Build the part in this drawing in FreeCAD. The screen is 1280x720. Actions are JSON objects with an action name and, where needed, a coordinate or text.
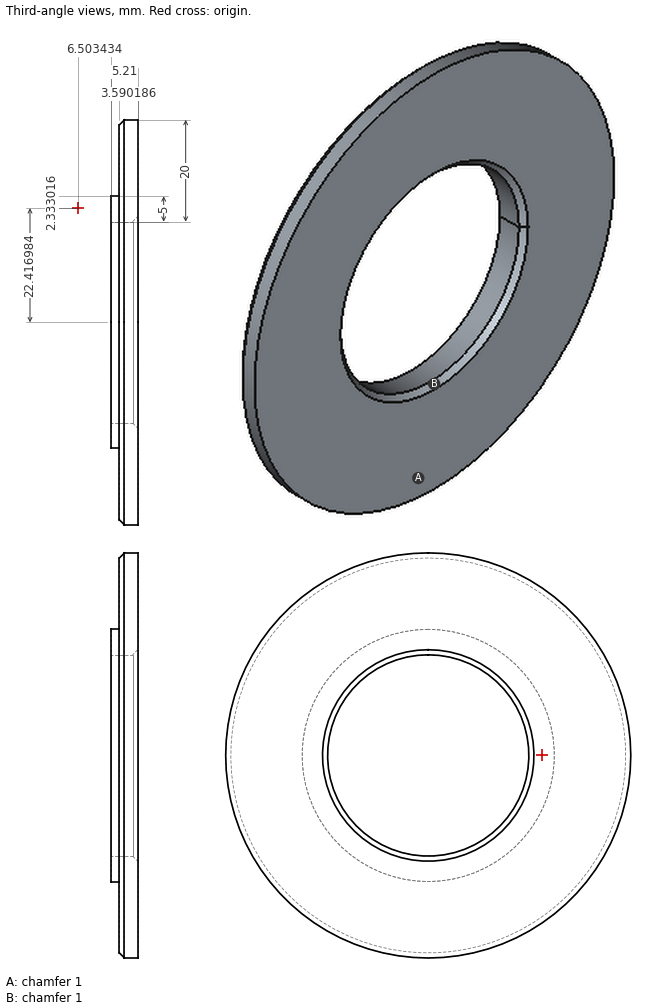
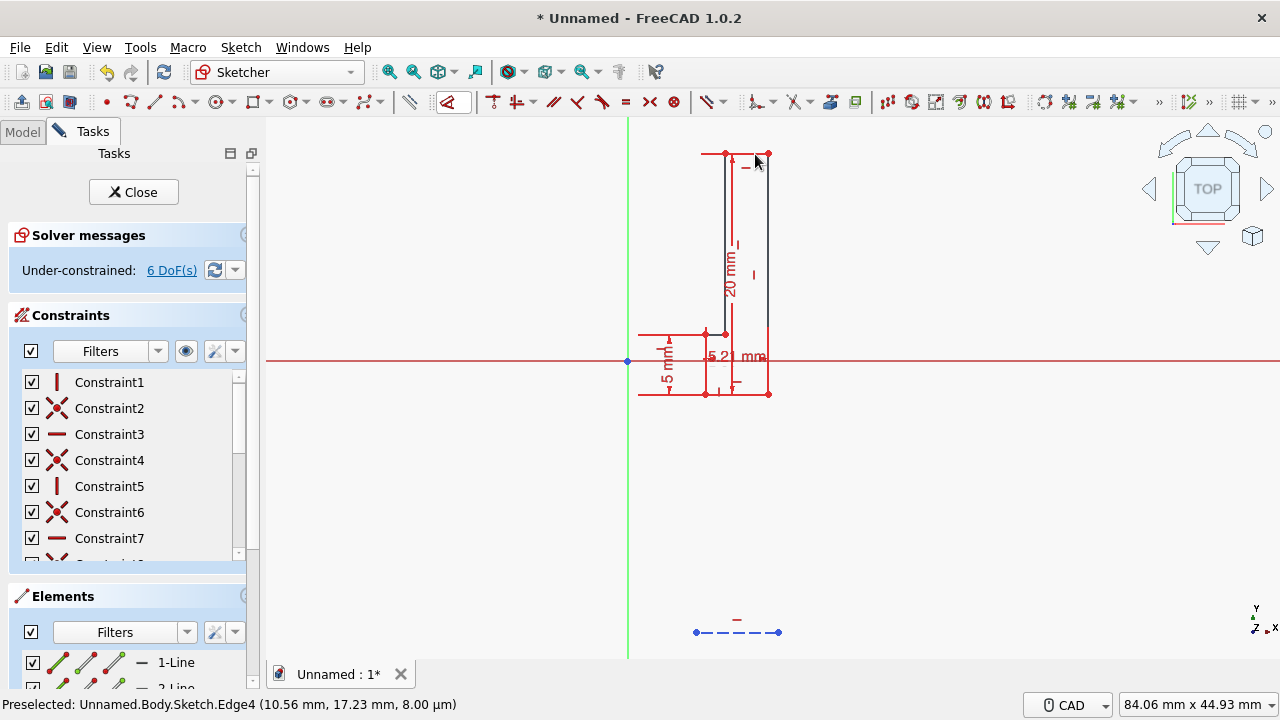
{"action": "key", "text": "l"}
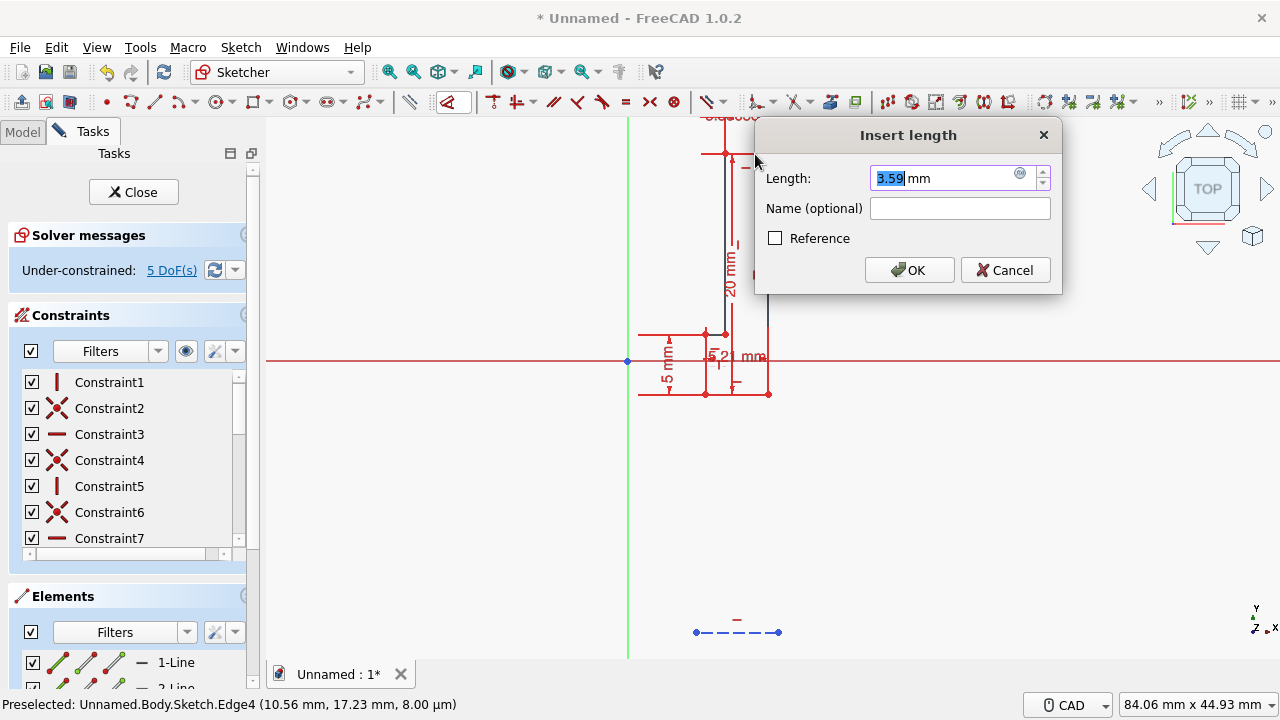
{"action": "type", "text": "3.590186"}
{"action": "key", "text": "Return"}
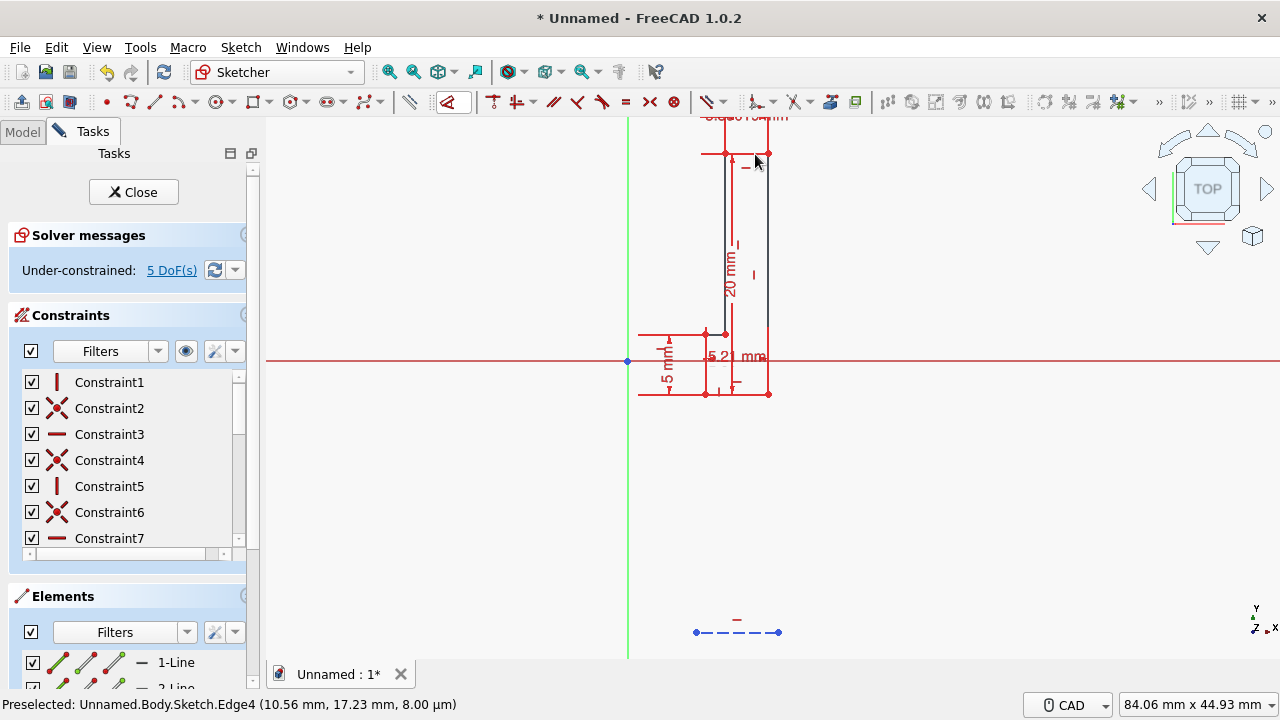
{"action": "left_click", "coordinate": [706, 334]}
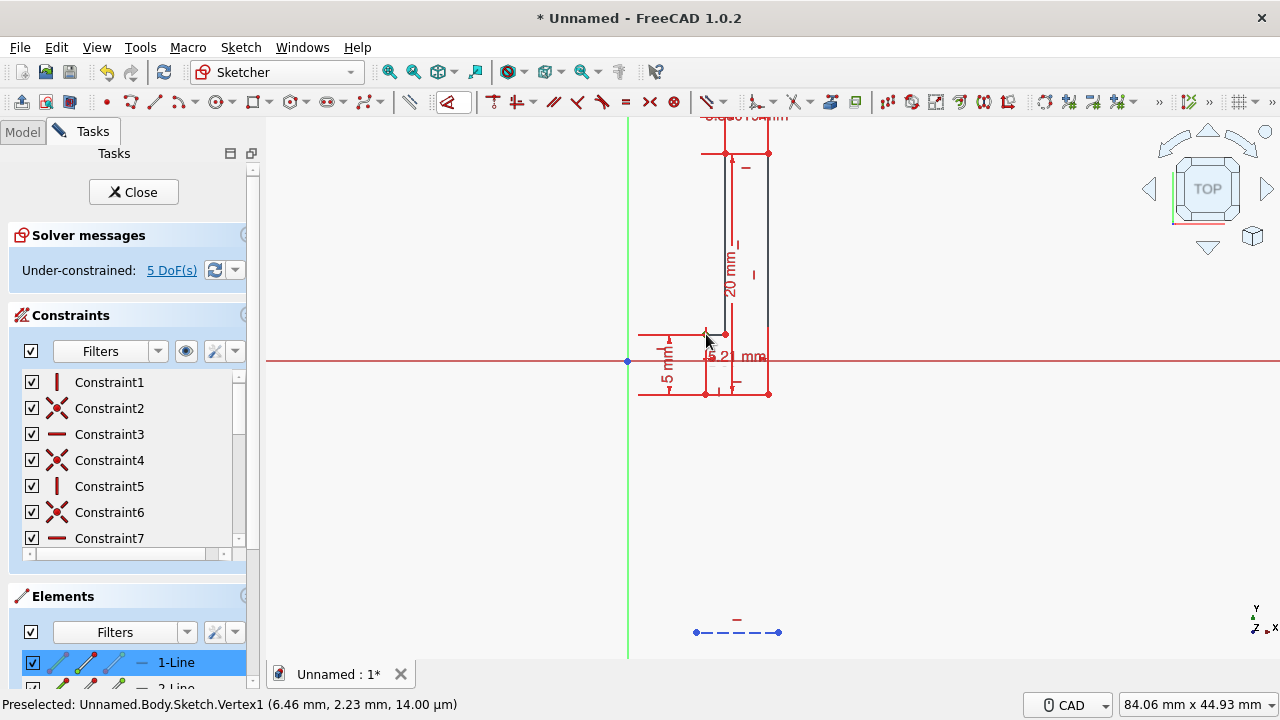
{"action": "key", "text": "l"}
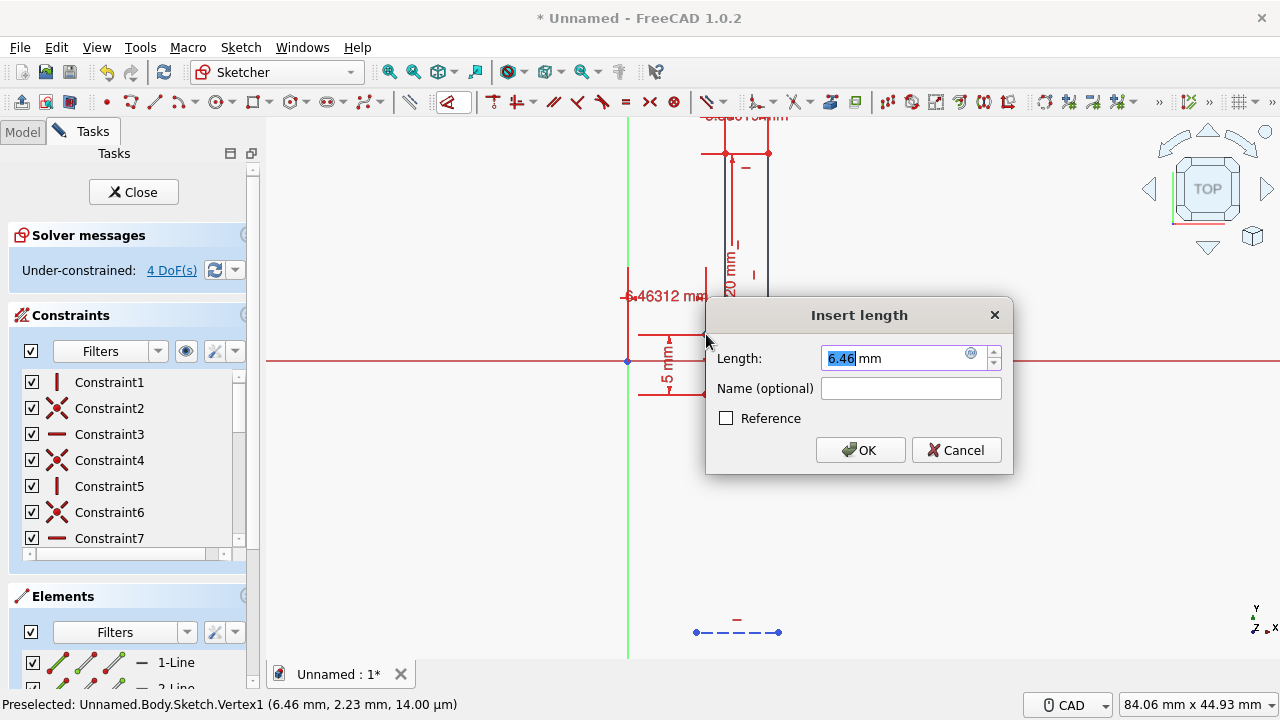
{"action": "type", "text": "6.503434"}
{"action": "key", "text": "Return"}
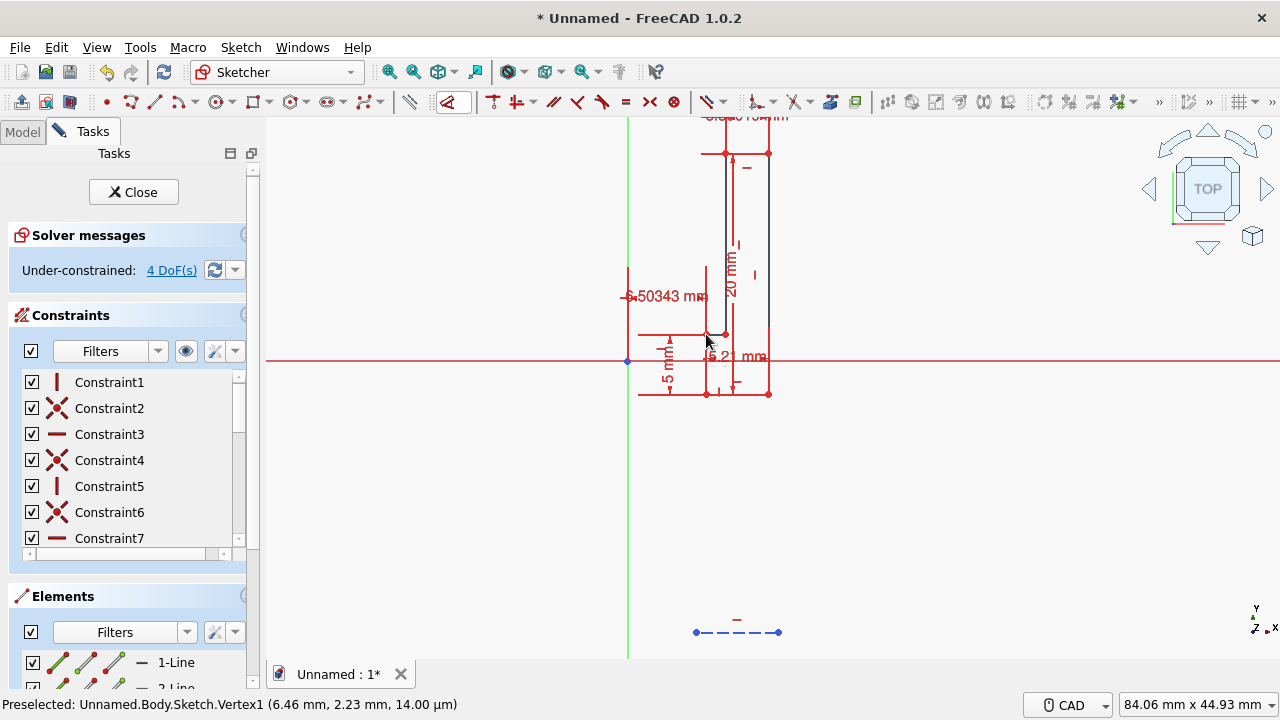
{"action": "scroll", "coordinate": [706, 334], "scroll_direction": "up", "scroll_amount": 2}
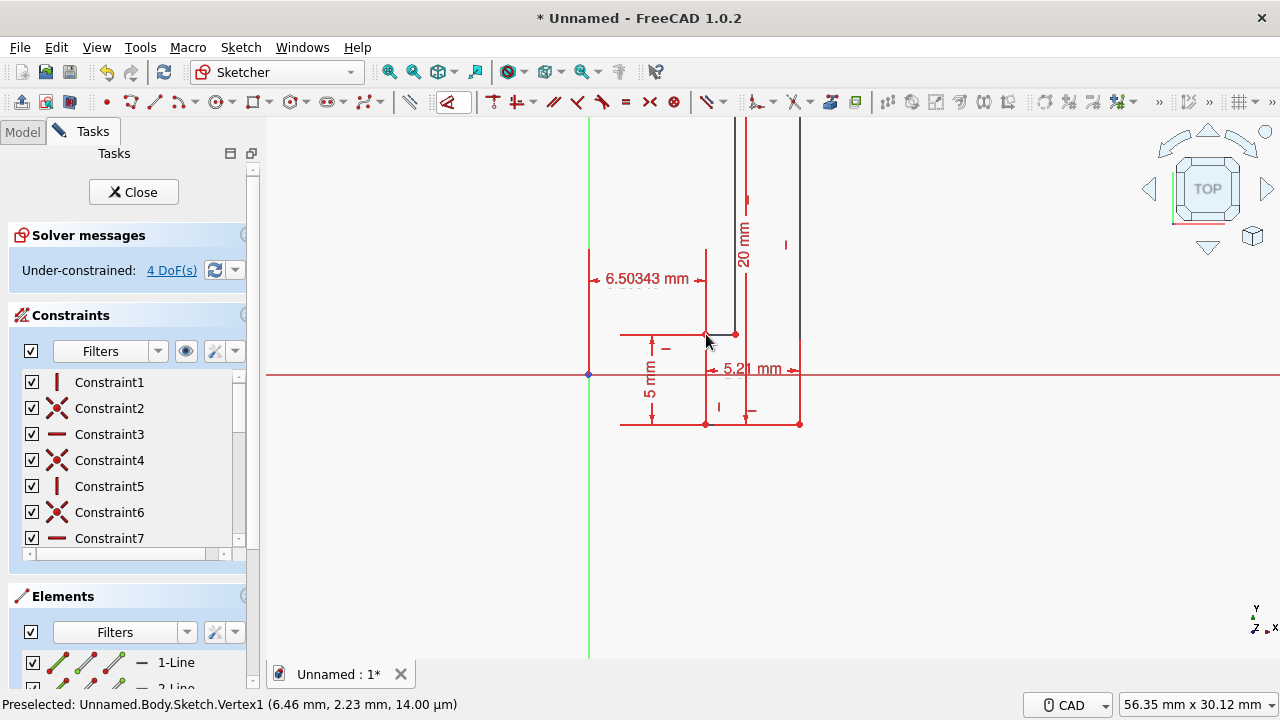
{"action": "left_click", "coordinate": [706, 335]}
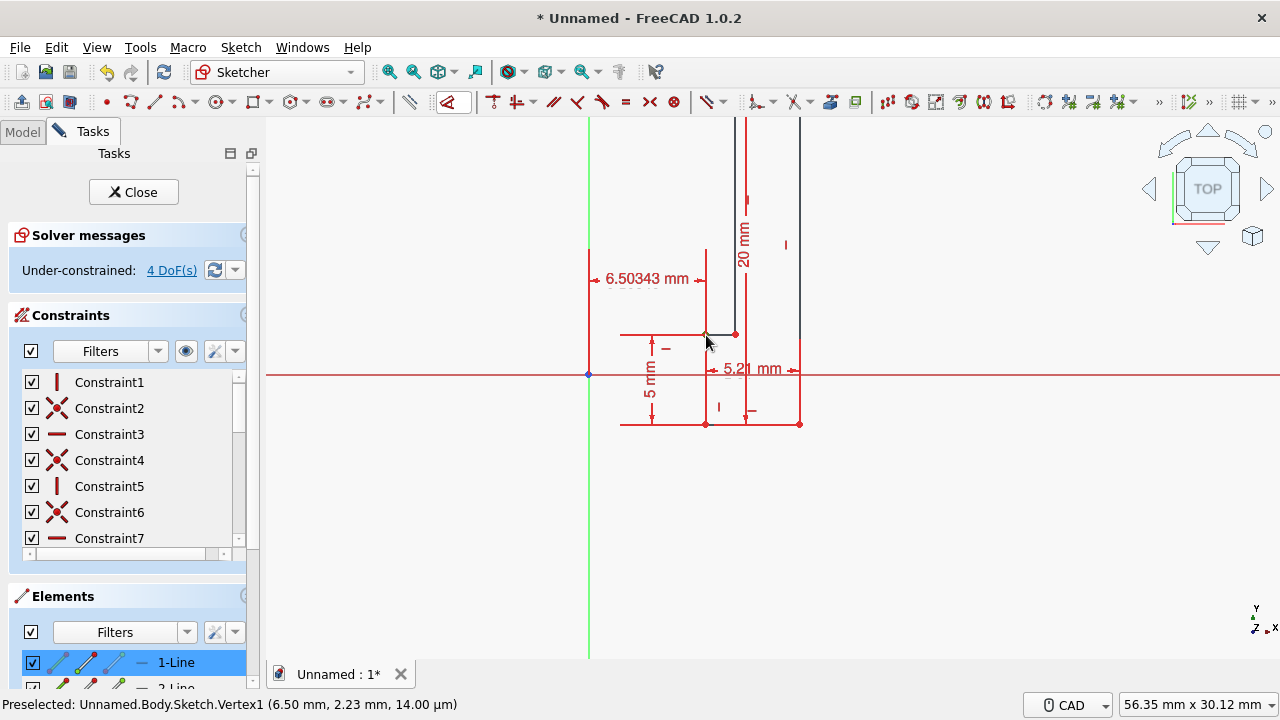
{"action": "key", "text": "i"}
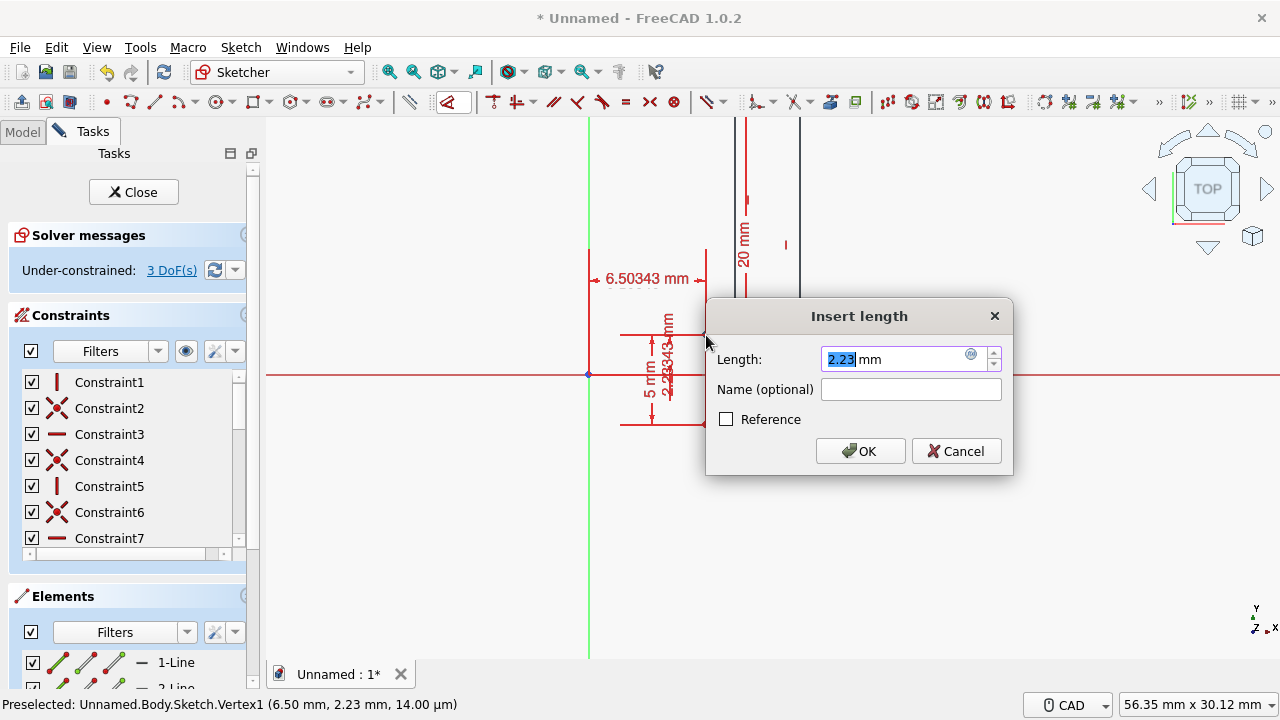
{"action": "type", "text": "2.333016"}
{"action": "key", "text": "Return"}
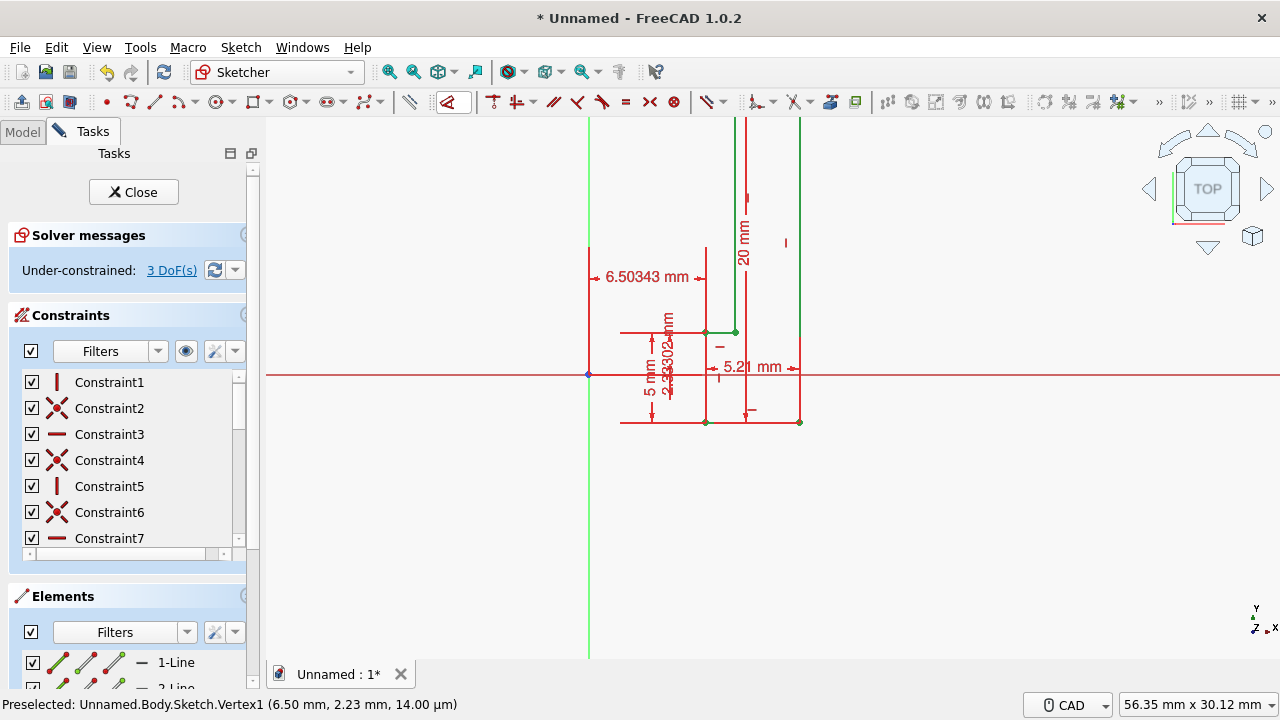
{"action": "scroll", "coordinate": [707, 361], "scroll_direction": "down", "scroll_amount": 4}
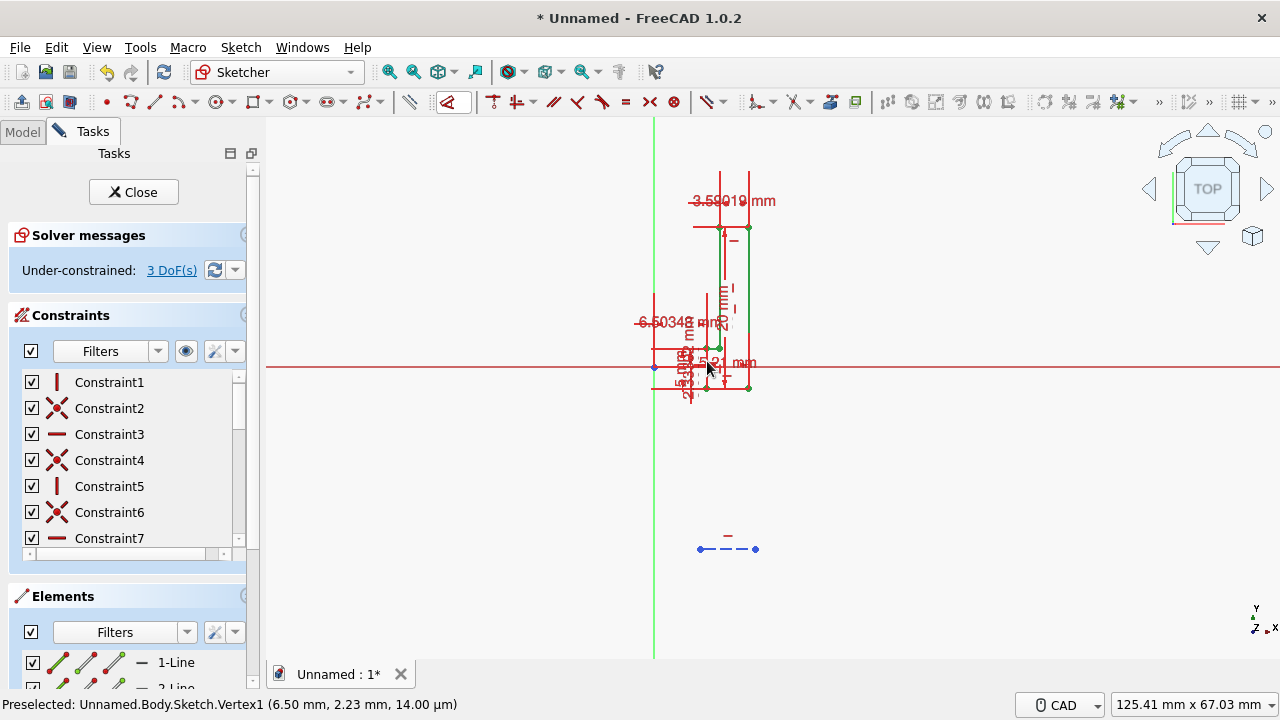
{"action": "left_click", "coordinate": [701, 549]}